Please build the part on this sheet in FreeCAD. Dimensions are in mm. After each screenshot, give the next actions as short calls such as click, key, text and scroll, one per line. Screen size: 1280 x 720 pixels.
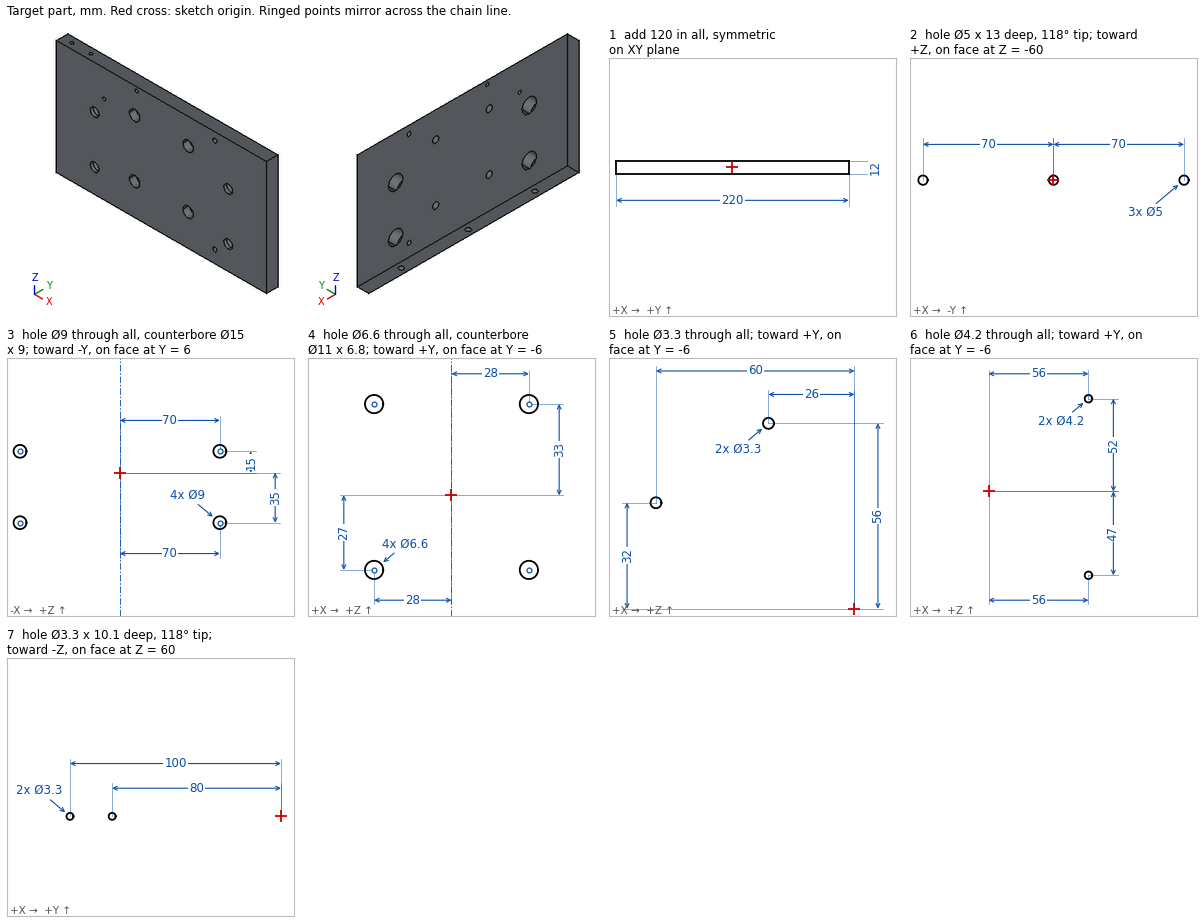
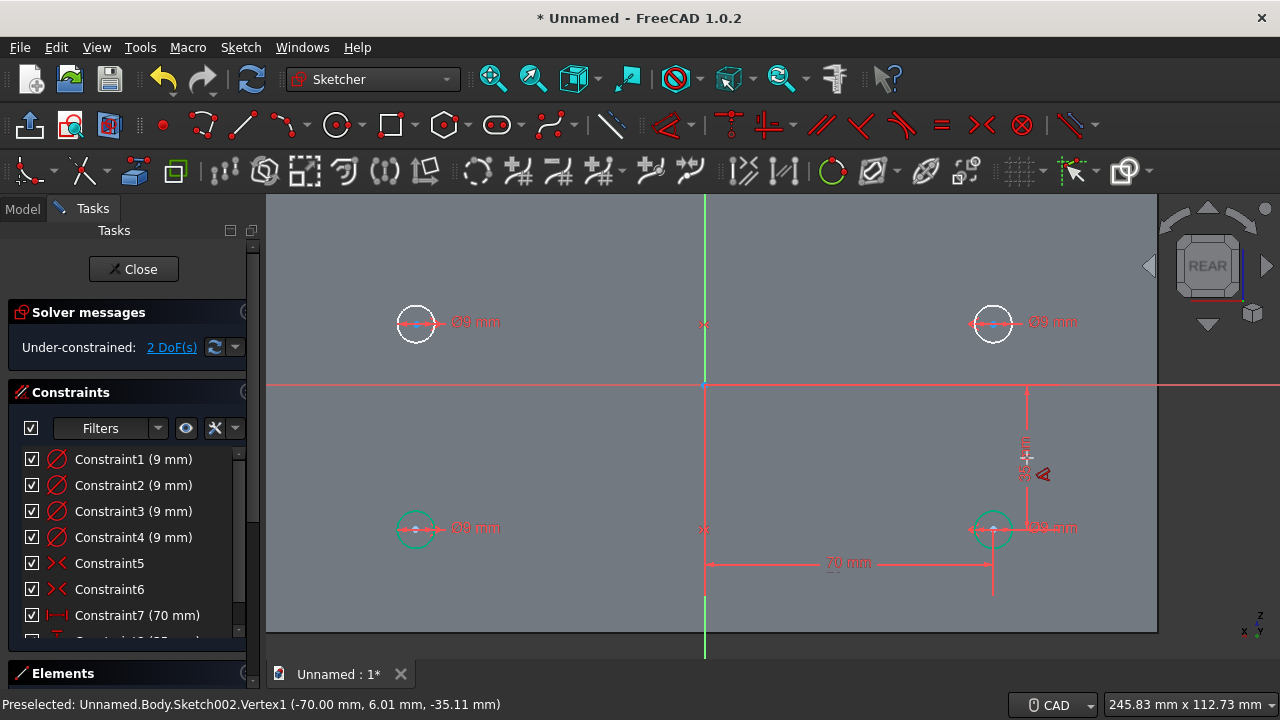
click(993, 324)
click(849, 290)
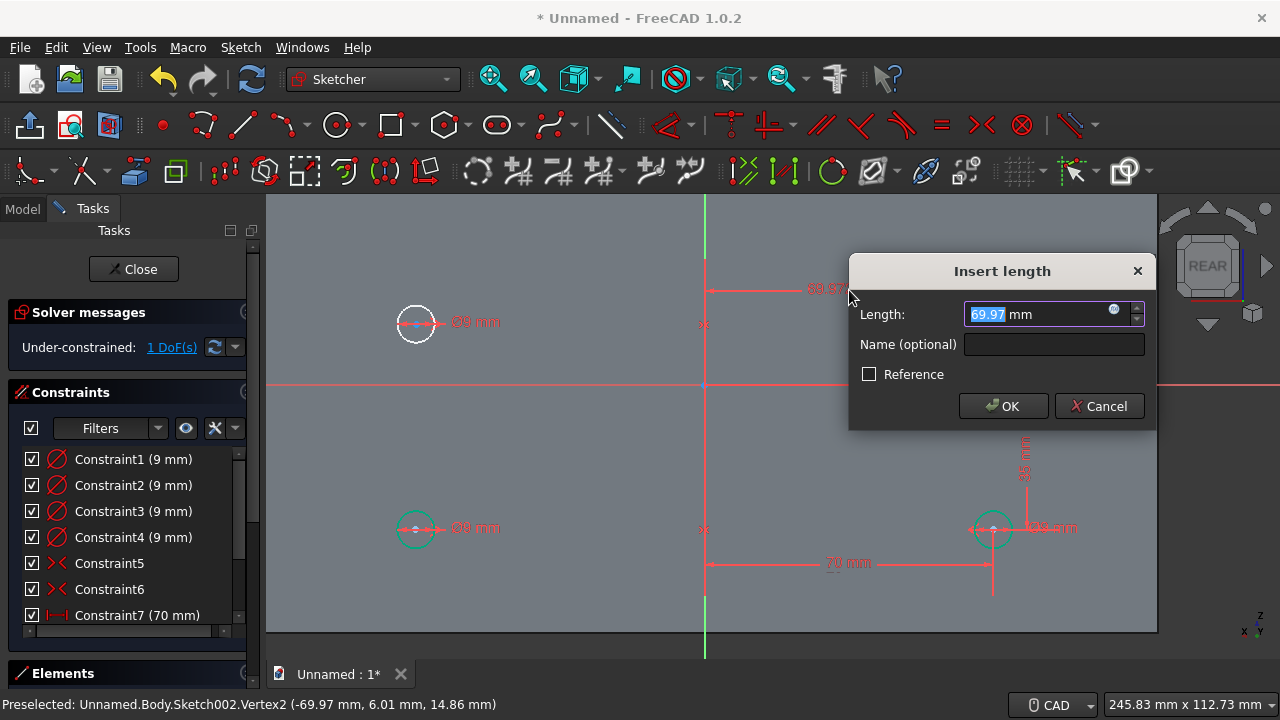
text(70)
key(Return)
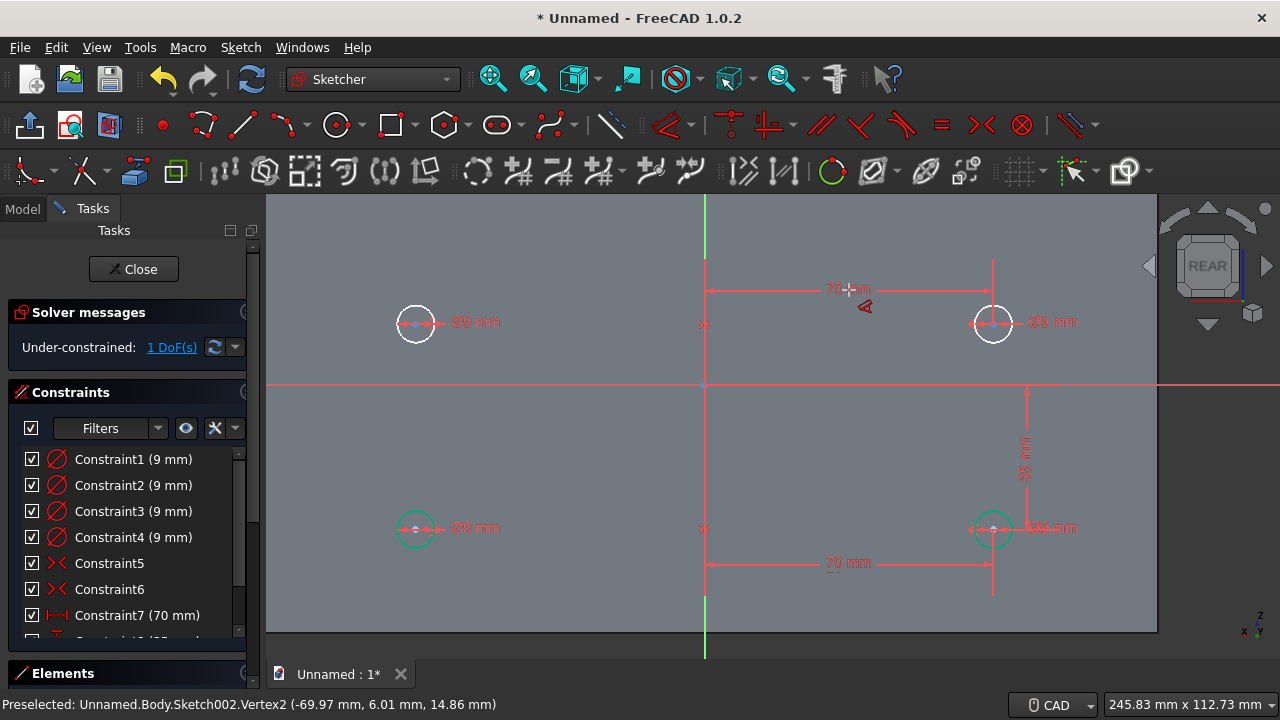
click(993, 324)
click(1027, 355)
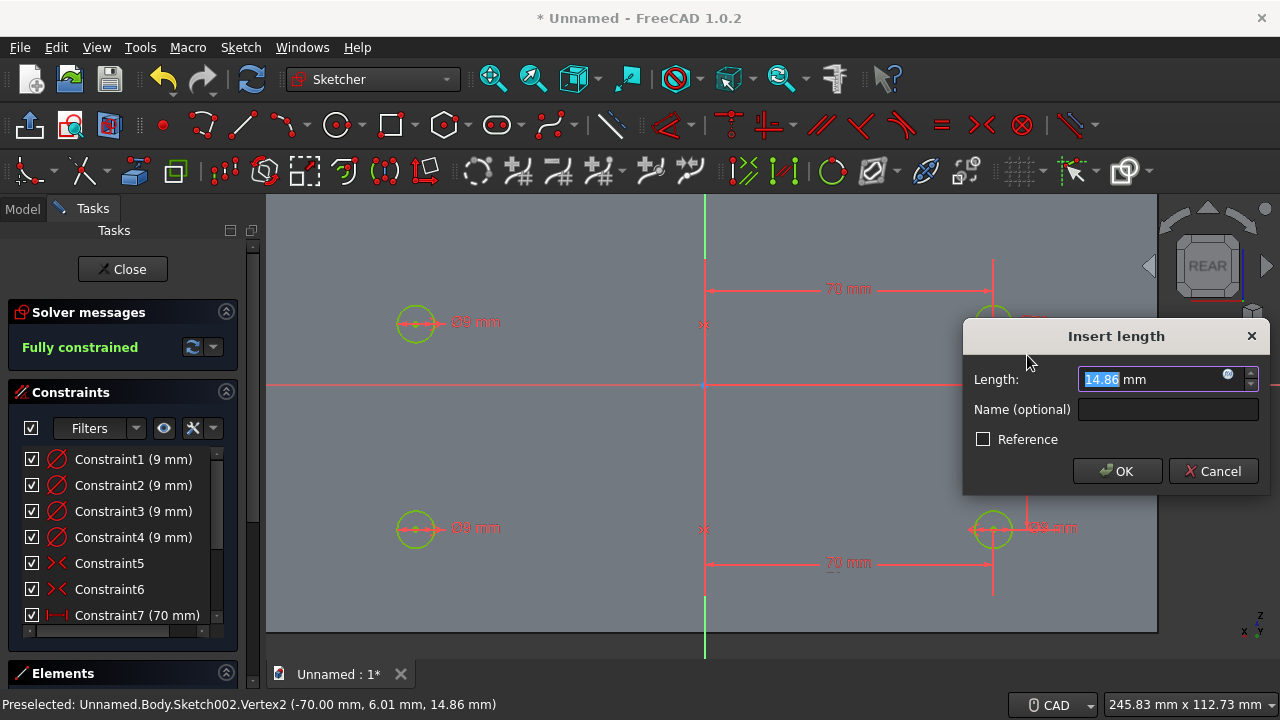
text(15)
key(Return)
key(Escape)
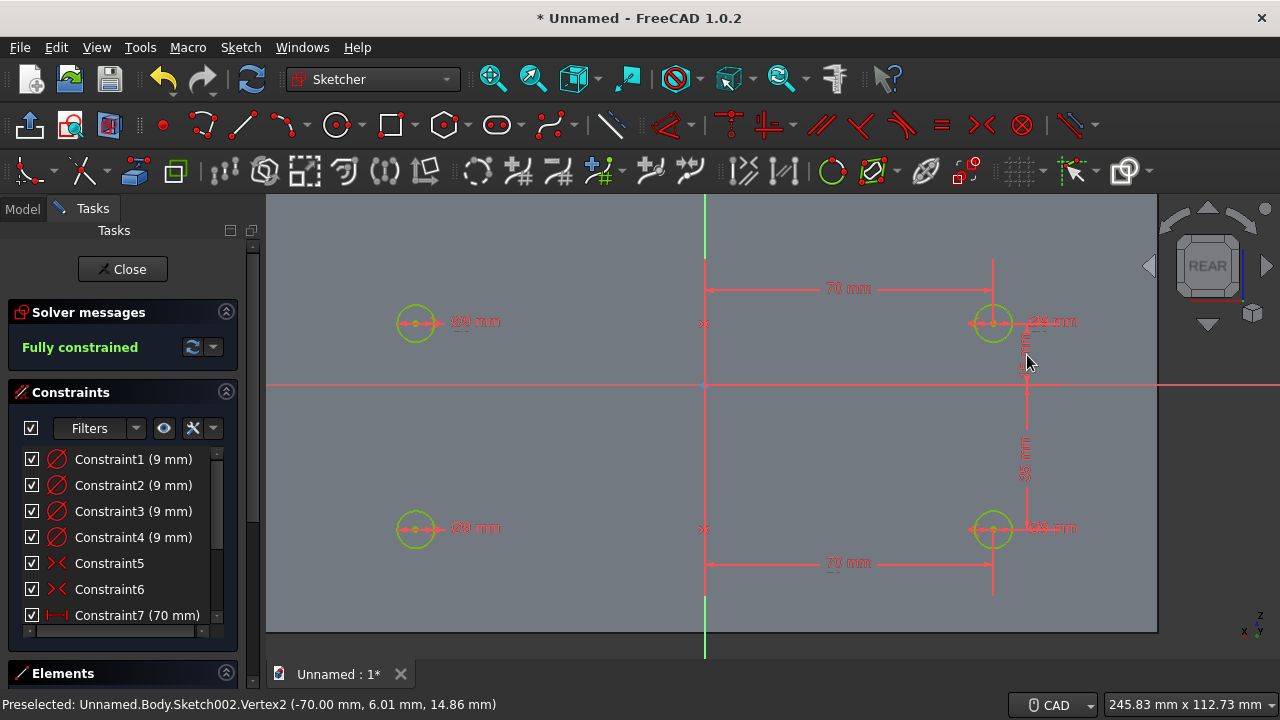
click(123, 269)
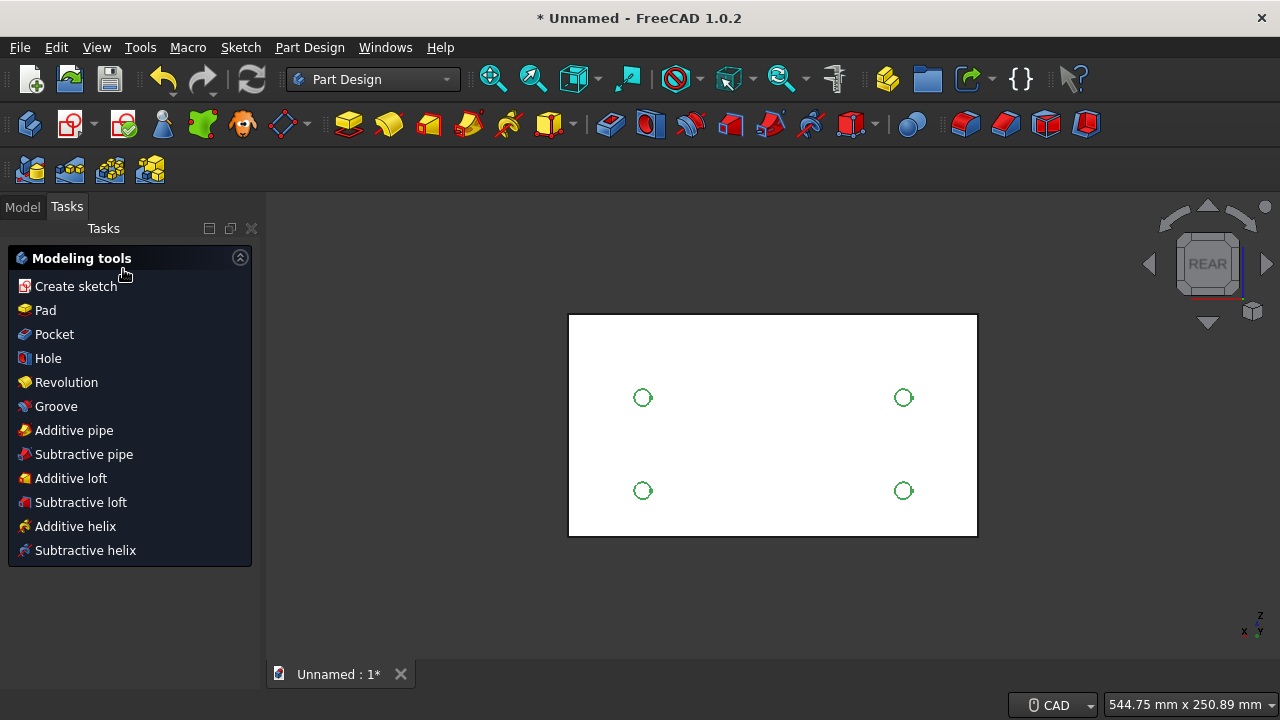
click(652, 124)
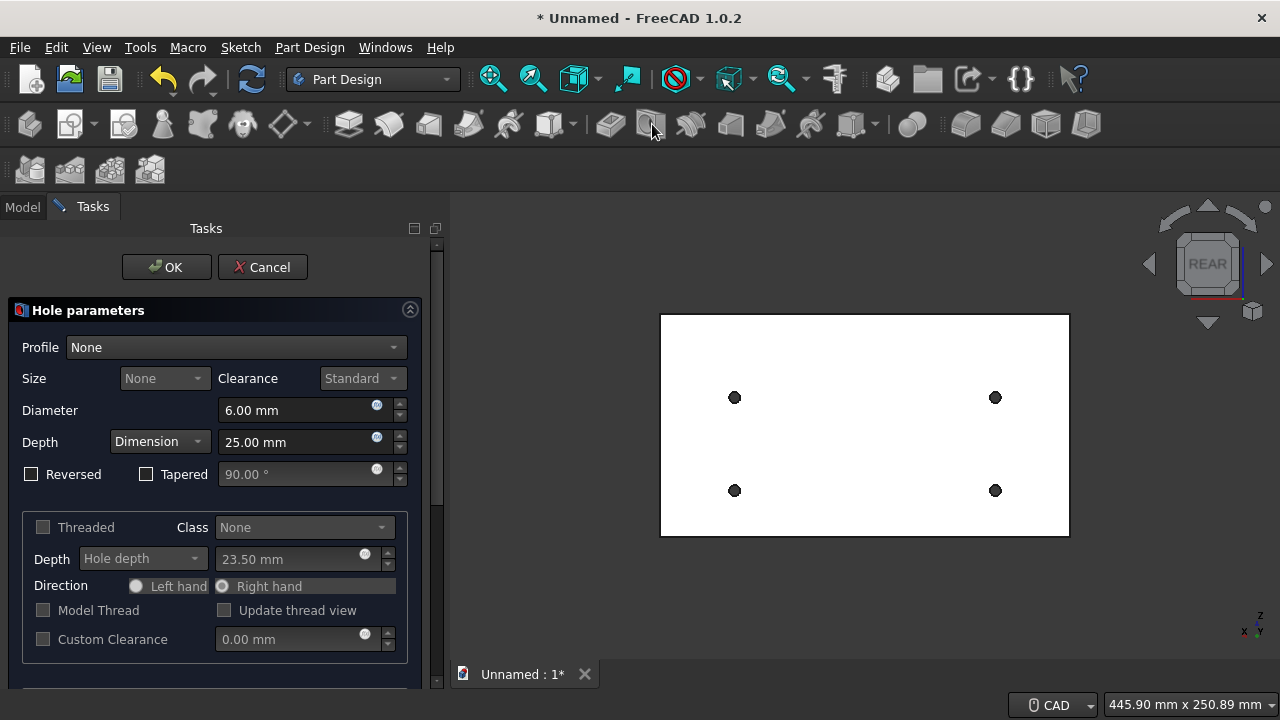
triple_click(305, 410)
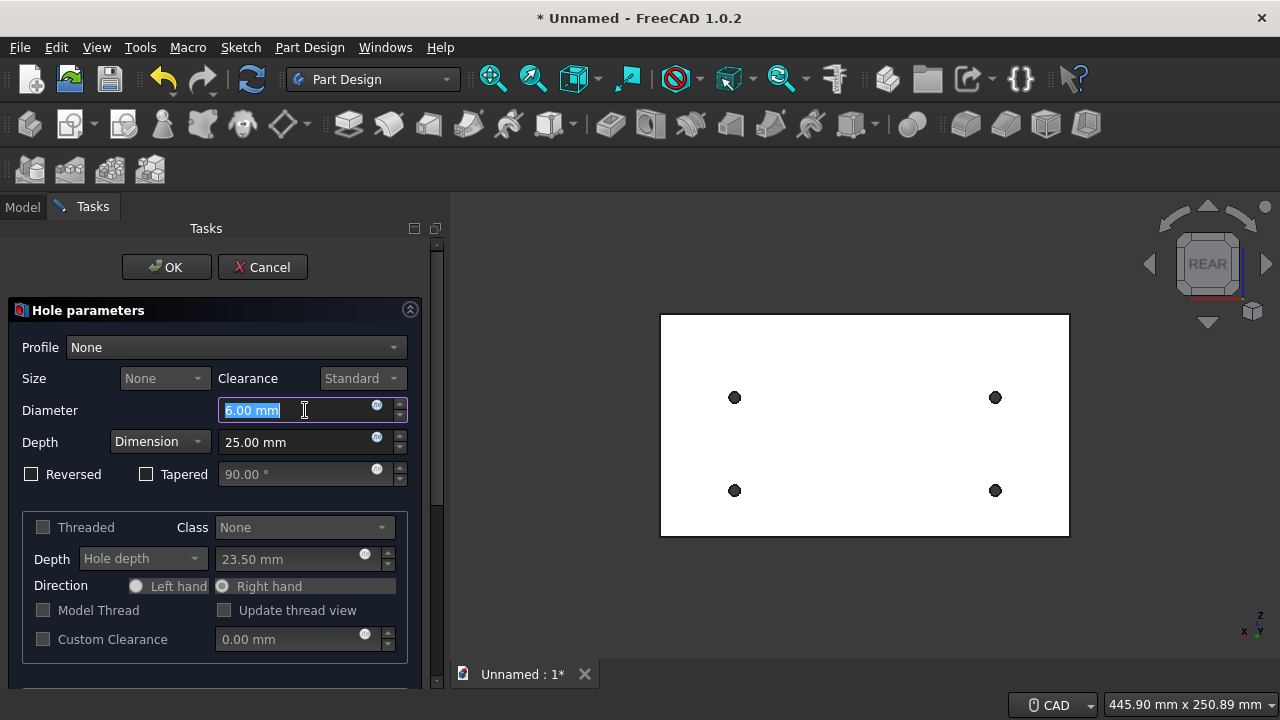
text(9)
key(Tab)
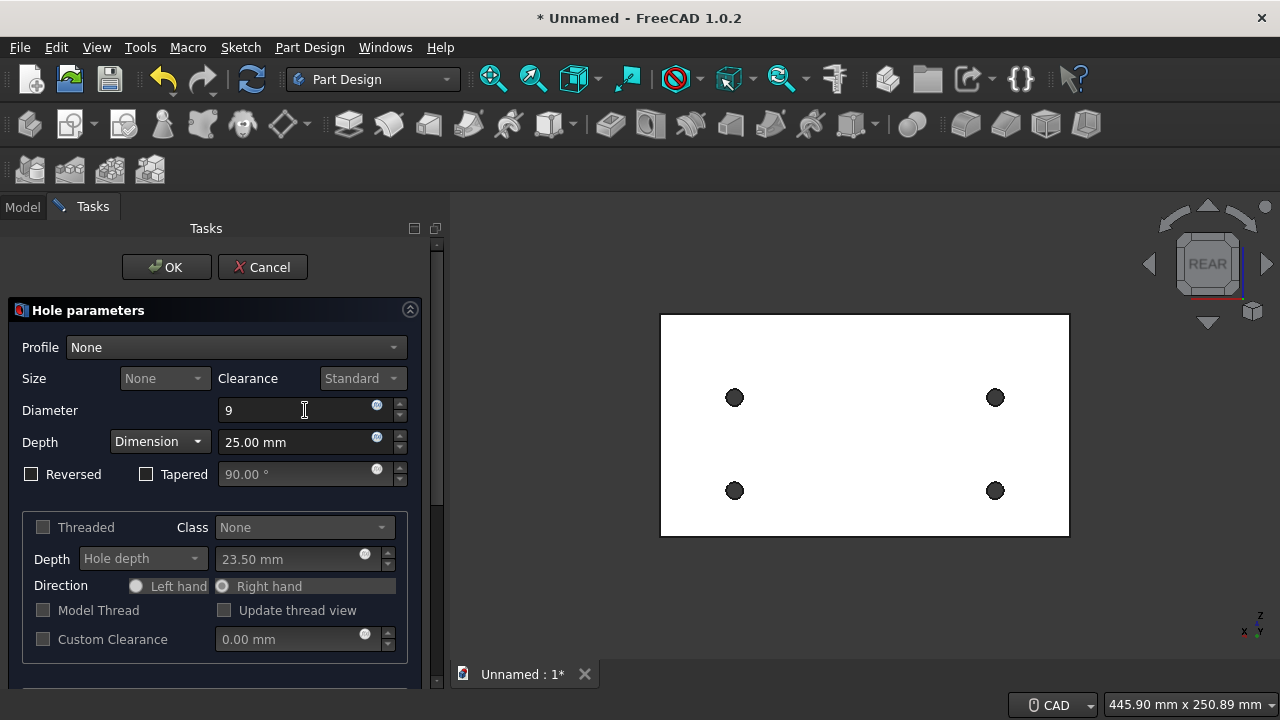
click(161, 442)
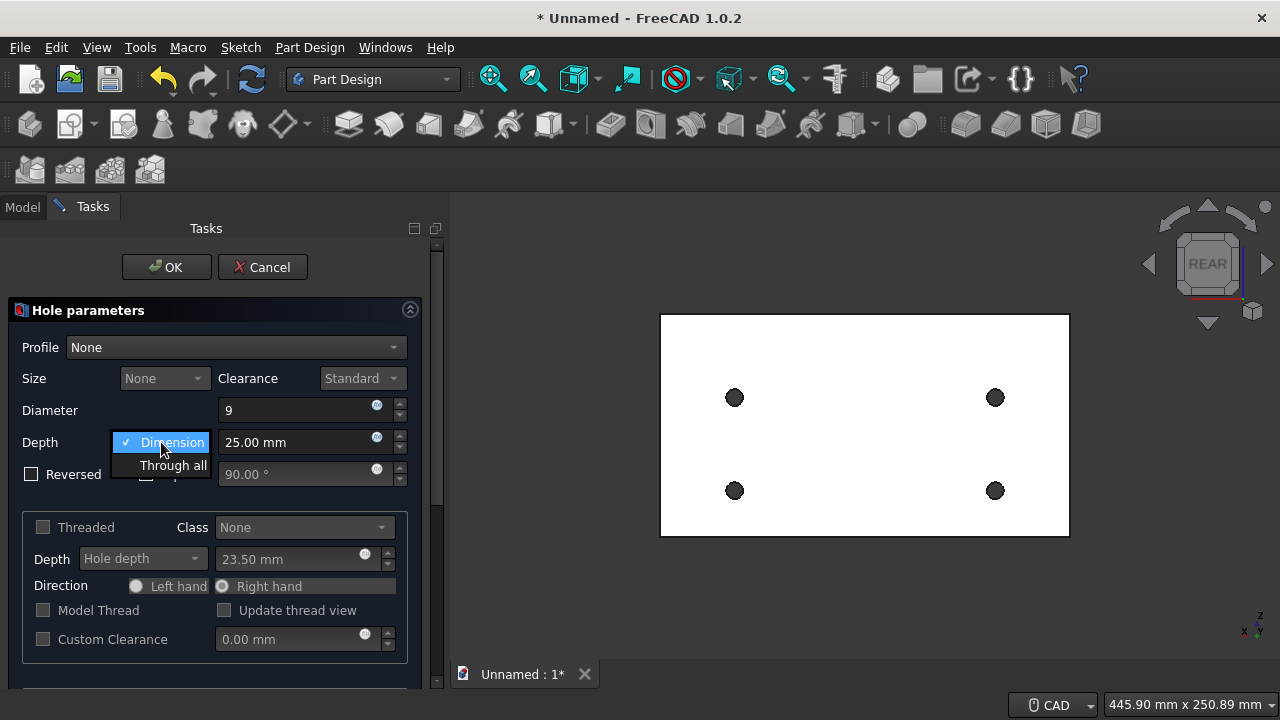
click(160, 466)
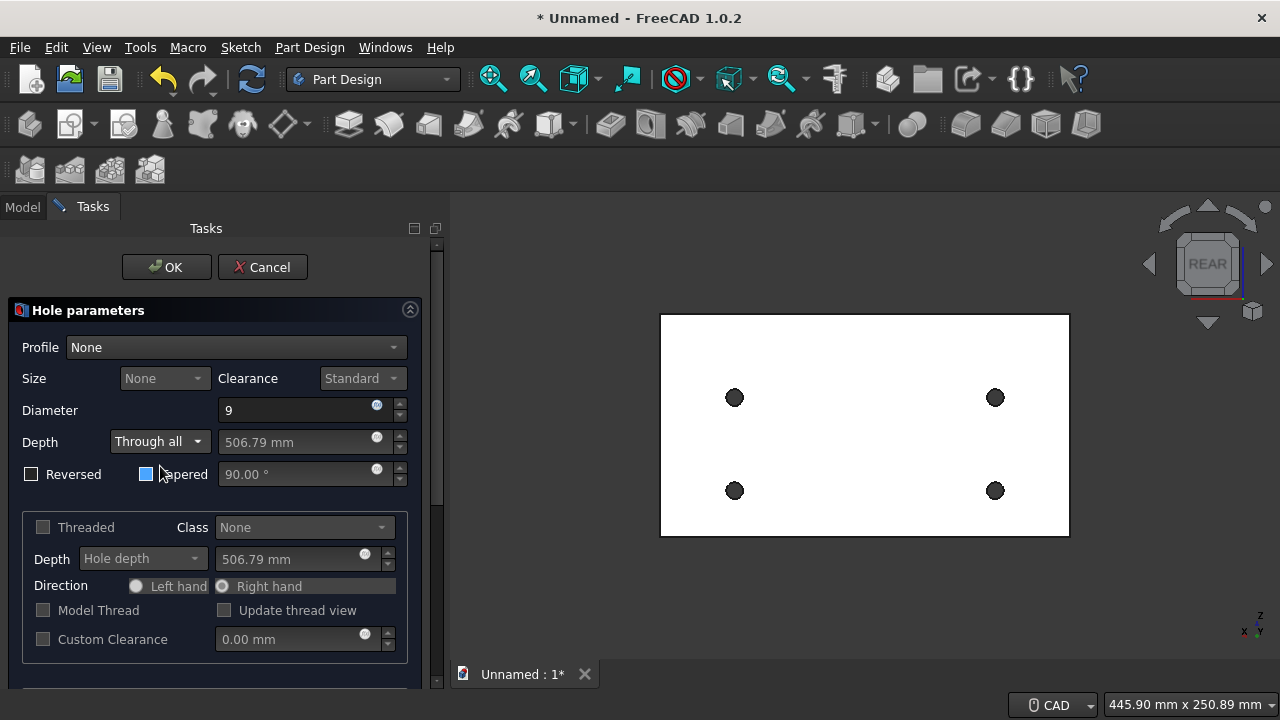
scroll(437, 463, down, 2)